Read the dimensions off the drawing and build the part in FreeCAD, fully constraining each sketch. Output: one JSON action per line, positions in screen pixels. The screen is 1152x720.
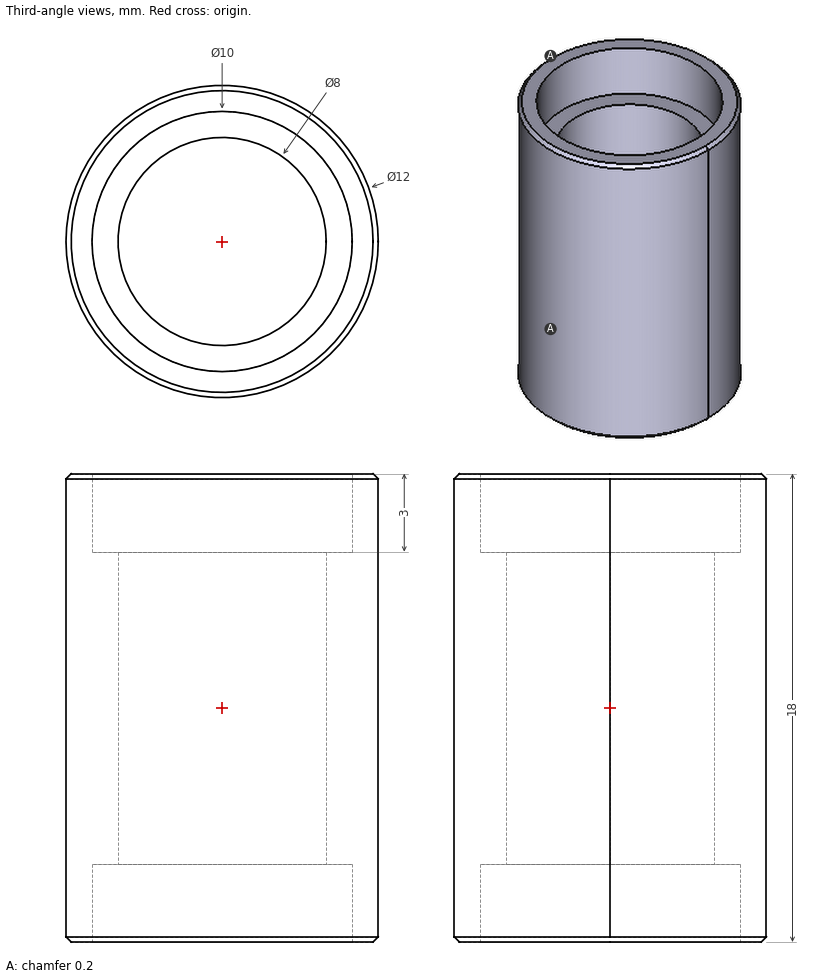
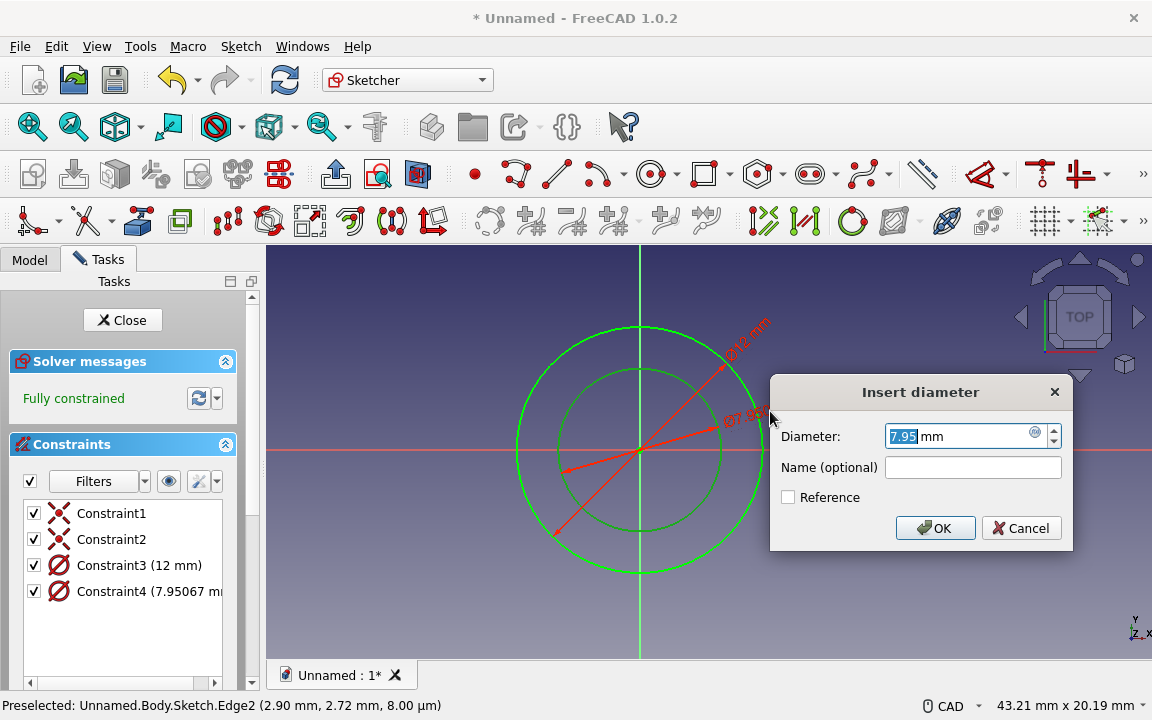
{"action": "type", "text": "8"}
{"action": "key", "text": "Return"}
{"action": "key", "text": "Escape"}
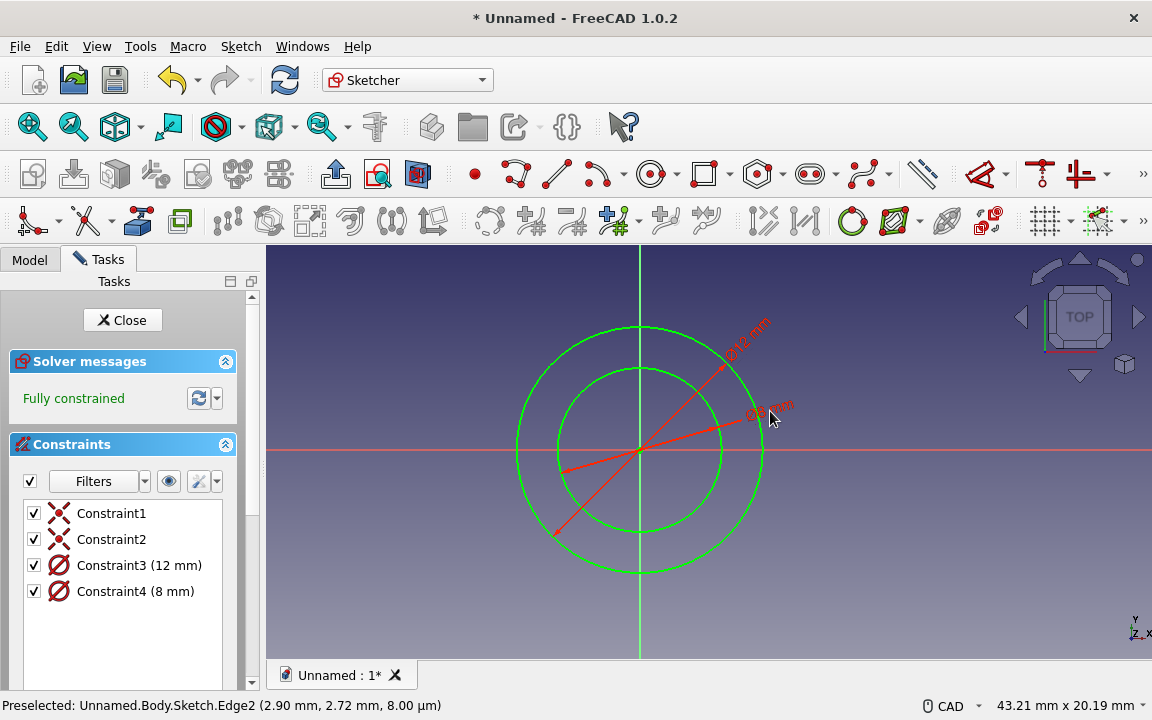
{"action": "left_click", "coordinate": [123, 320]}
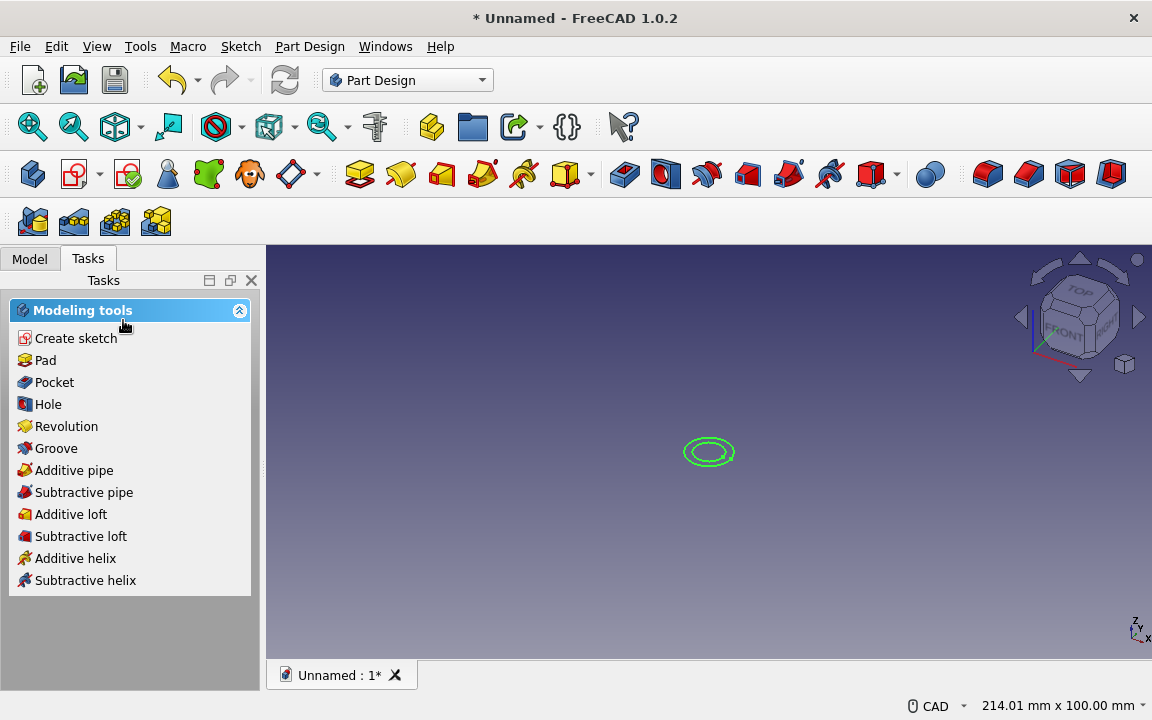
{"action": "left_click", "coordinate": [360, 174]}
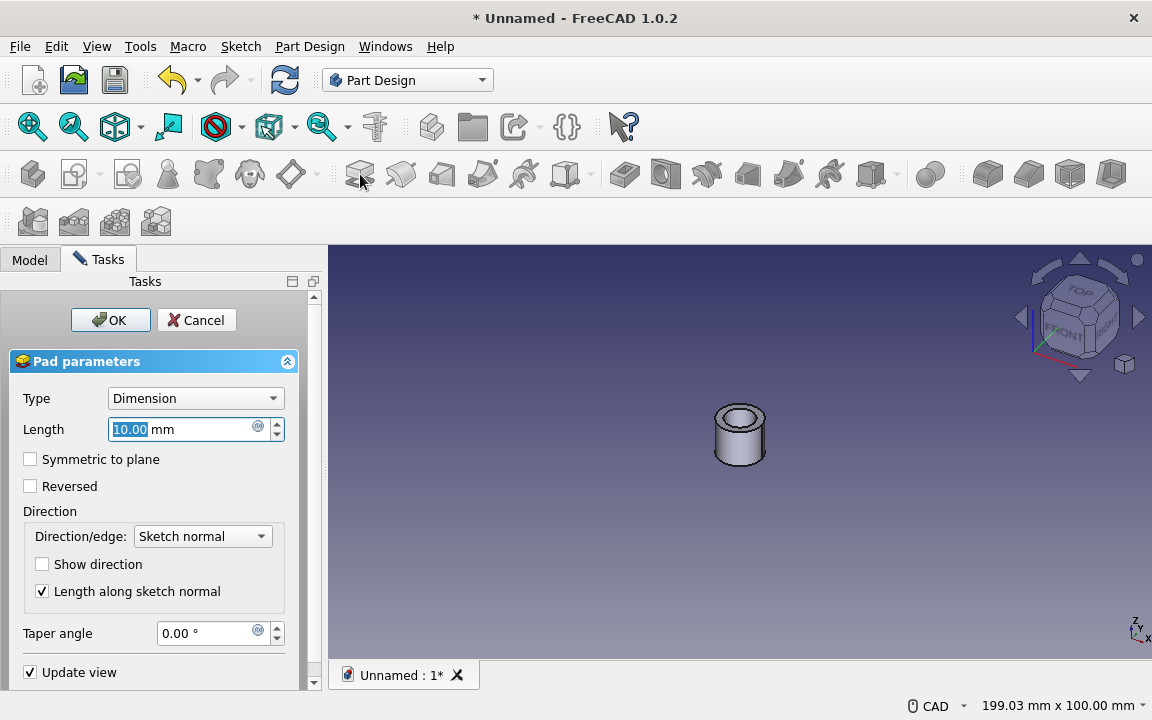
{"action": "type", "text": "18"}
{"action": "key", "text": "Tab"}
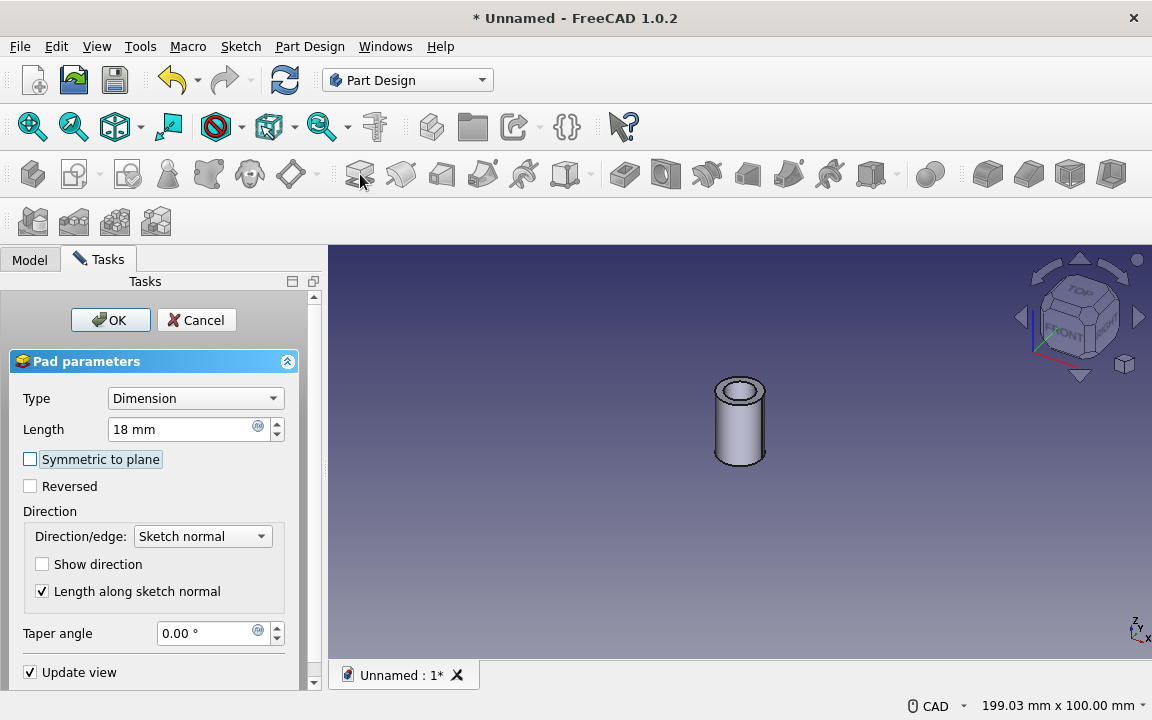
{"action": "left_click", "coordinate": [31, 459]}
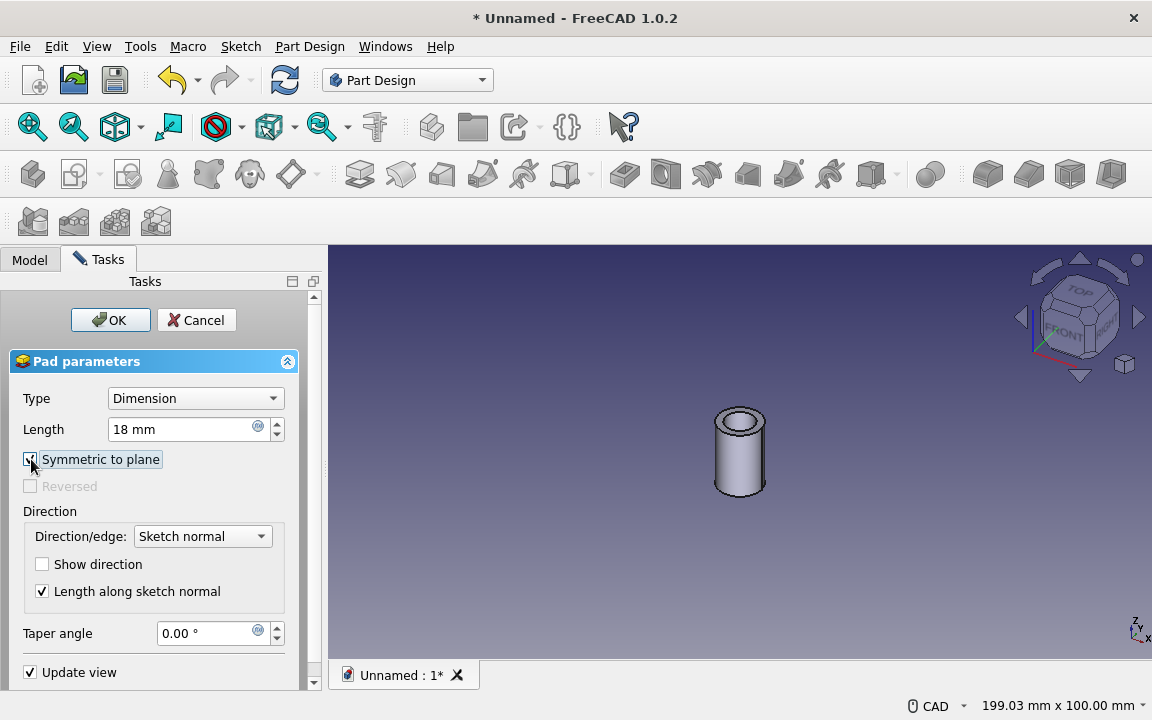
{"action": "left_click", "coordinate": [111, 320]}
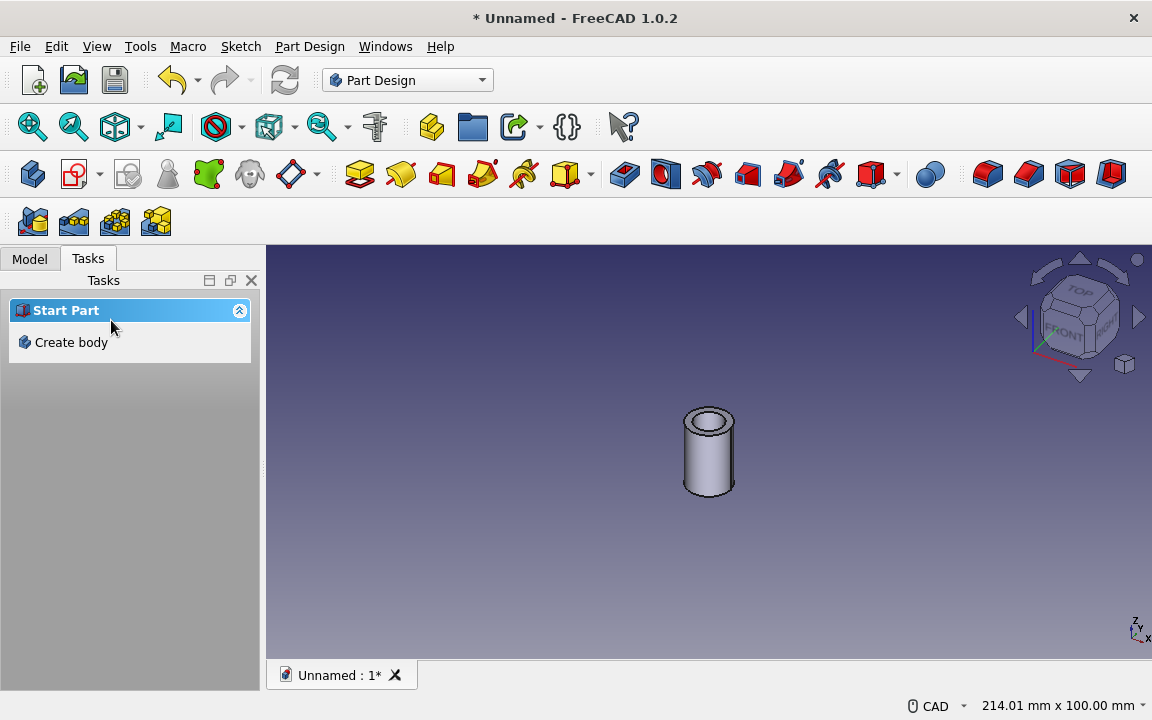
{"action": "left_click", "coordinate": [33, 128]}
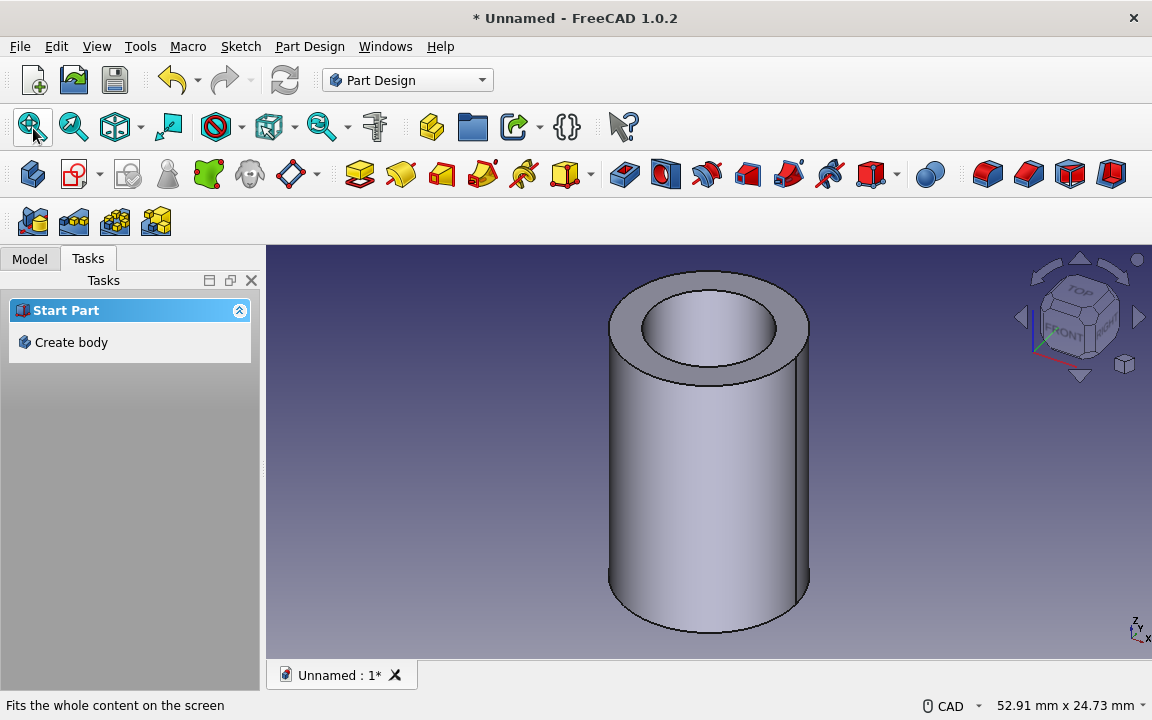
{"action": "left_click", "coordinate": [784, 352]}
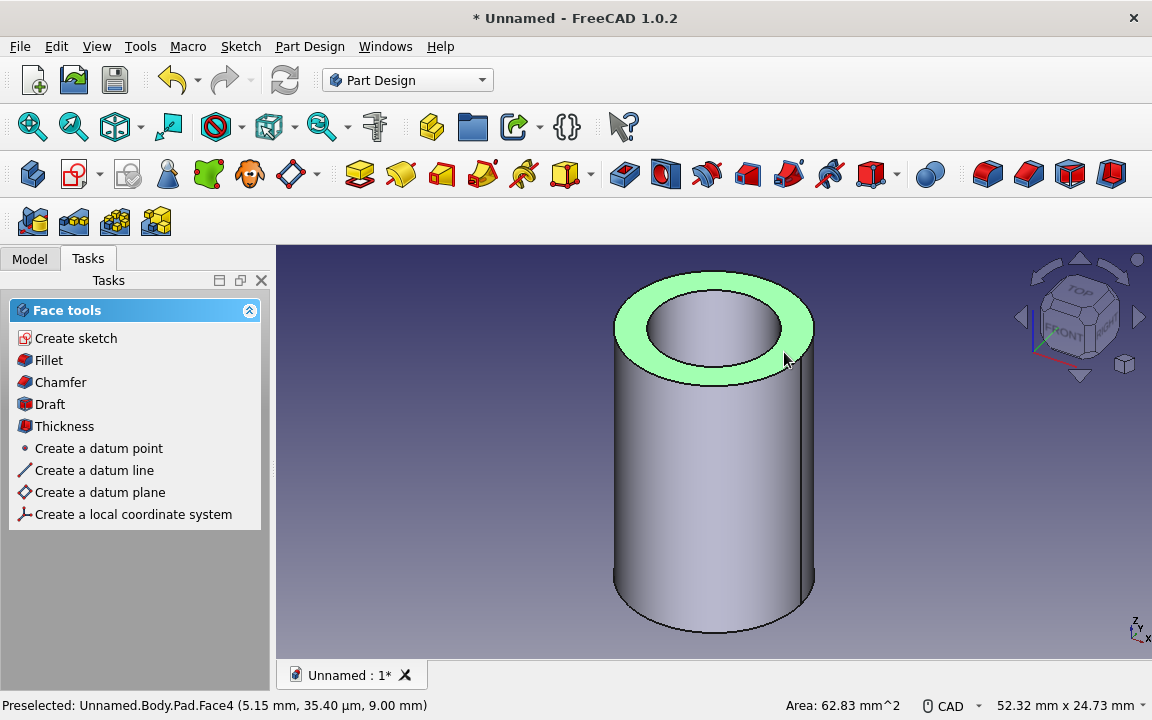
{"action": "left_click", "coordinate": [74, 174]}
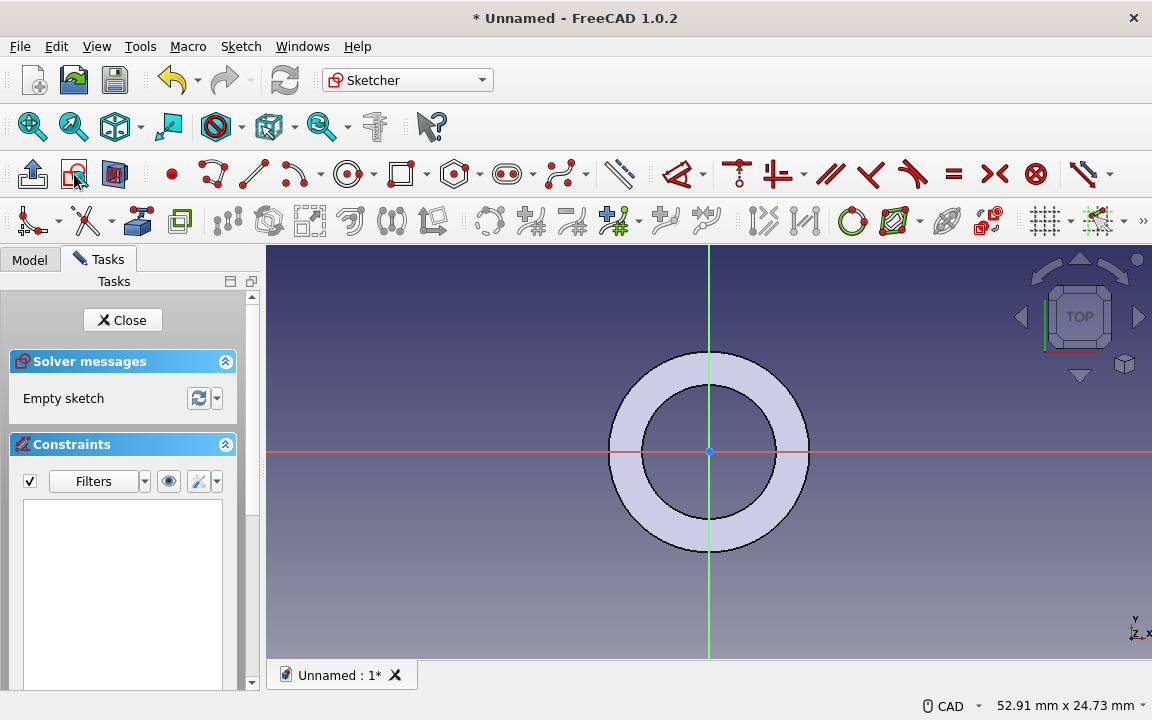
{"action": "scroll", "coordinate": [848, 452], "scroll_direction": "up", "scroll_amount": 2}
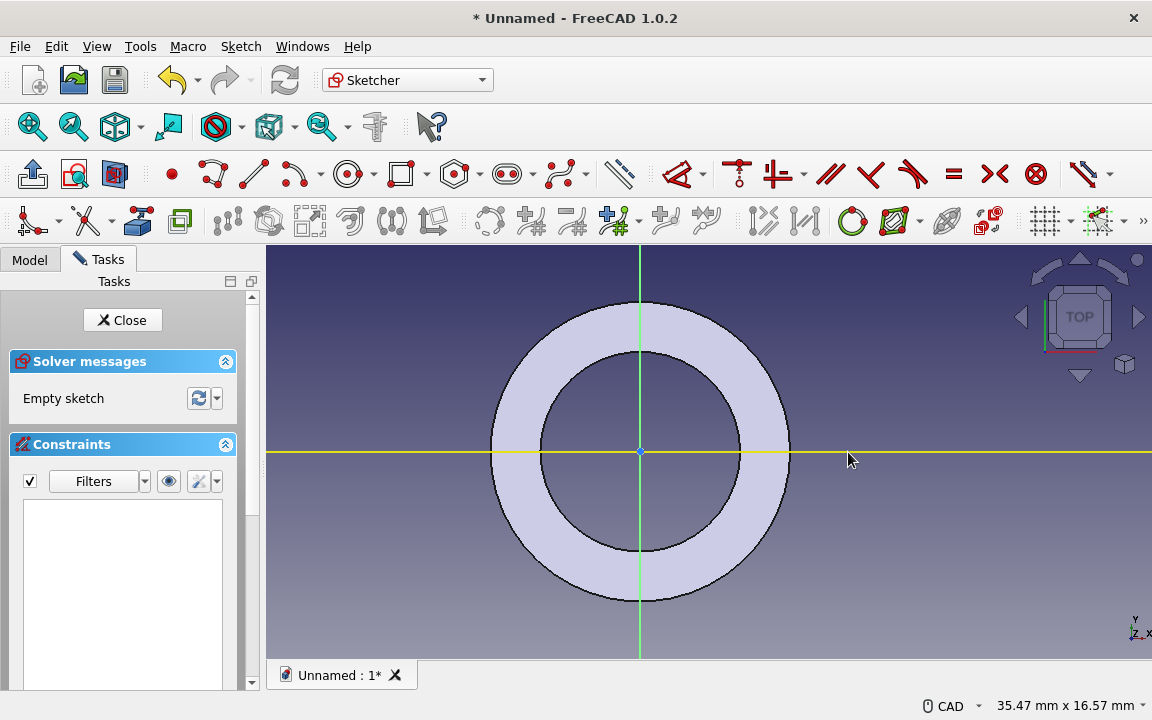
{"action": "left_click", "coordinate": [348, 174]}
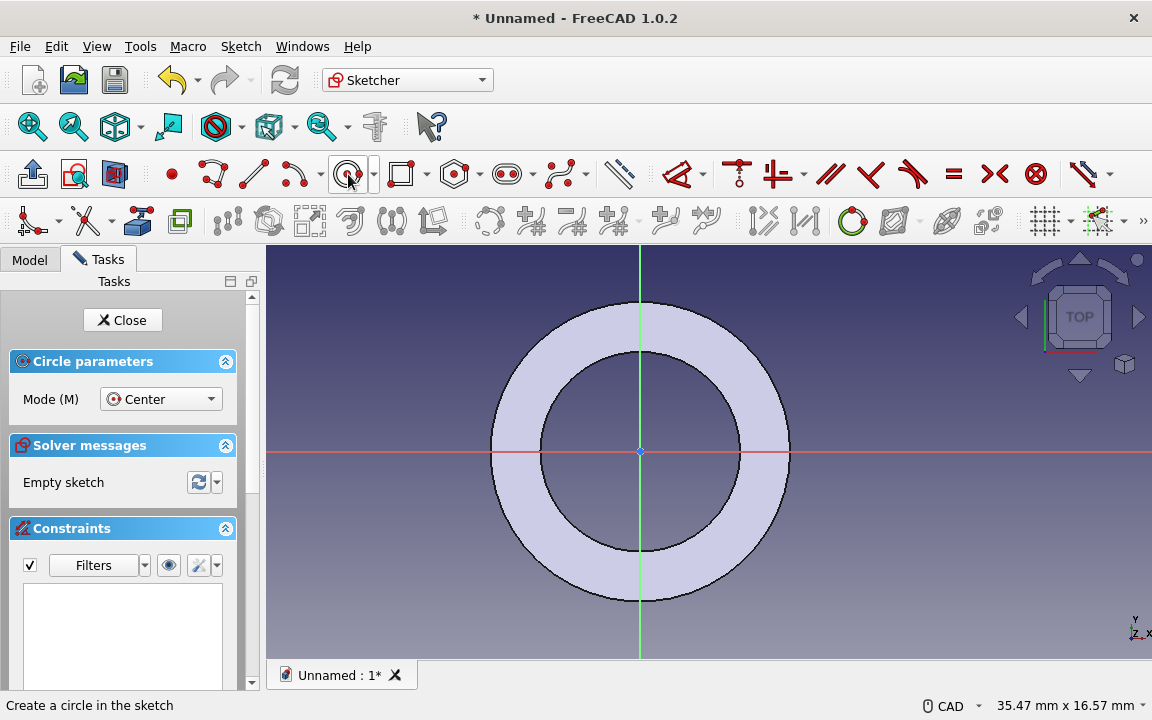
{"action": "left_click", "coordinate": [640, 452]}
{"action": "left_click", "coordinate": [729, 363]}
{"action": "key", "text": "Escape"}